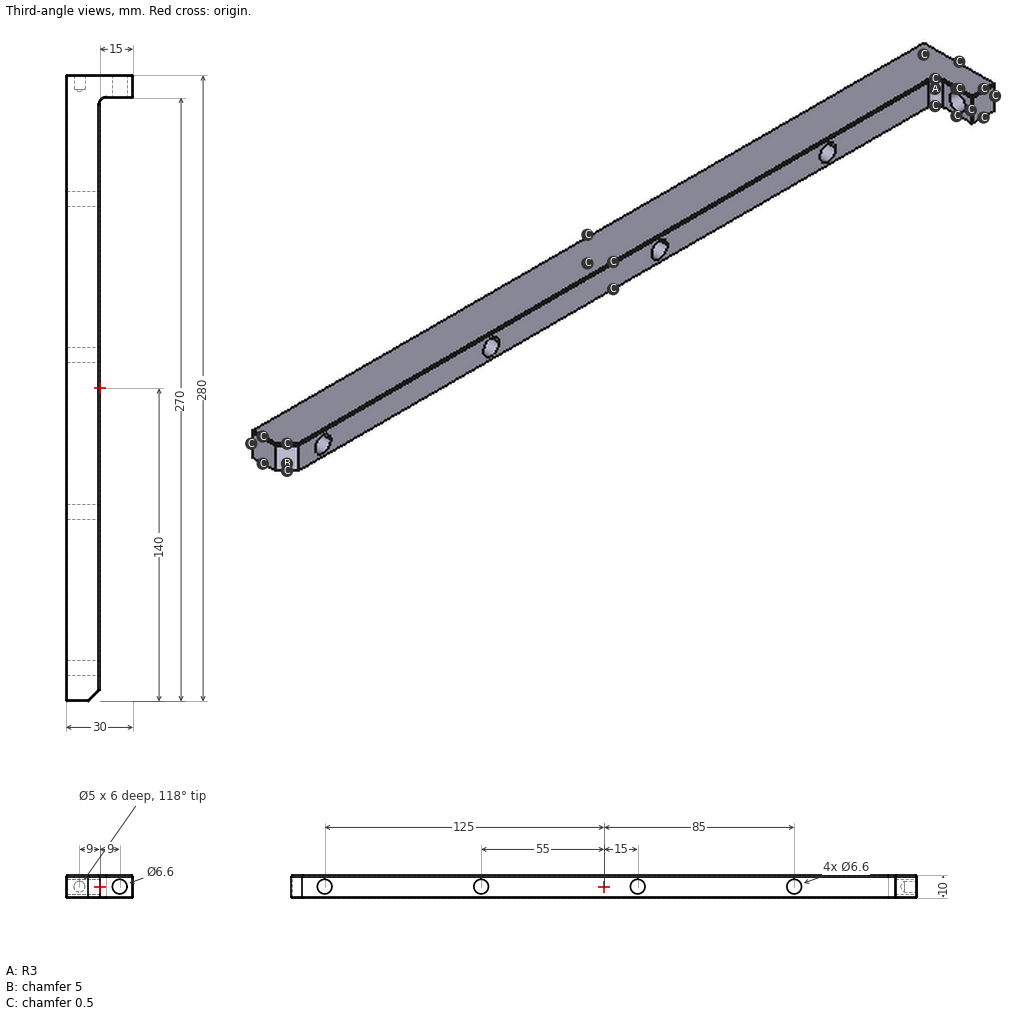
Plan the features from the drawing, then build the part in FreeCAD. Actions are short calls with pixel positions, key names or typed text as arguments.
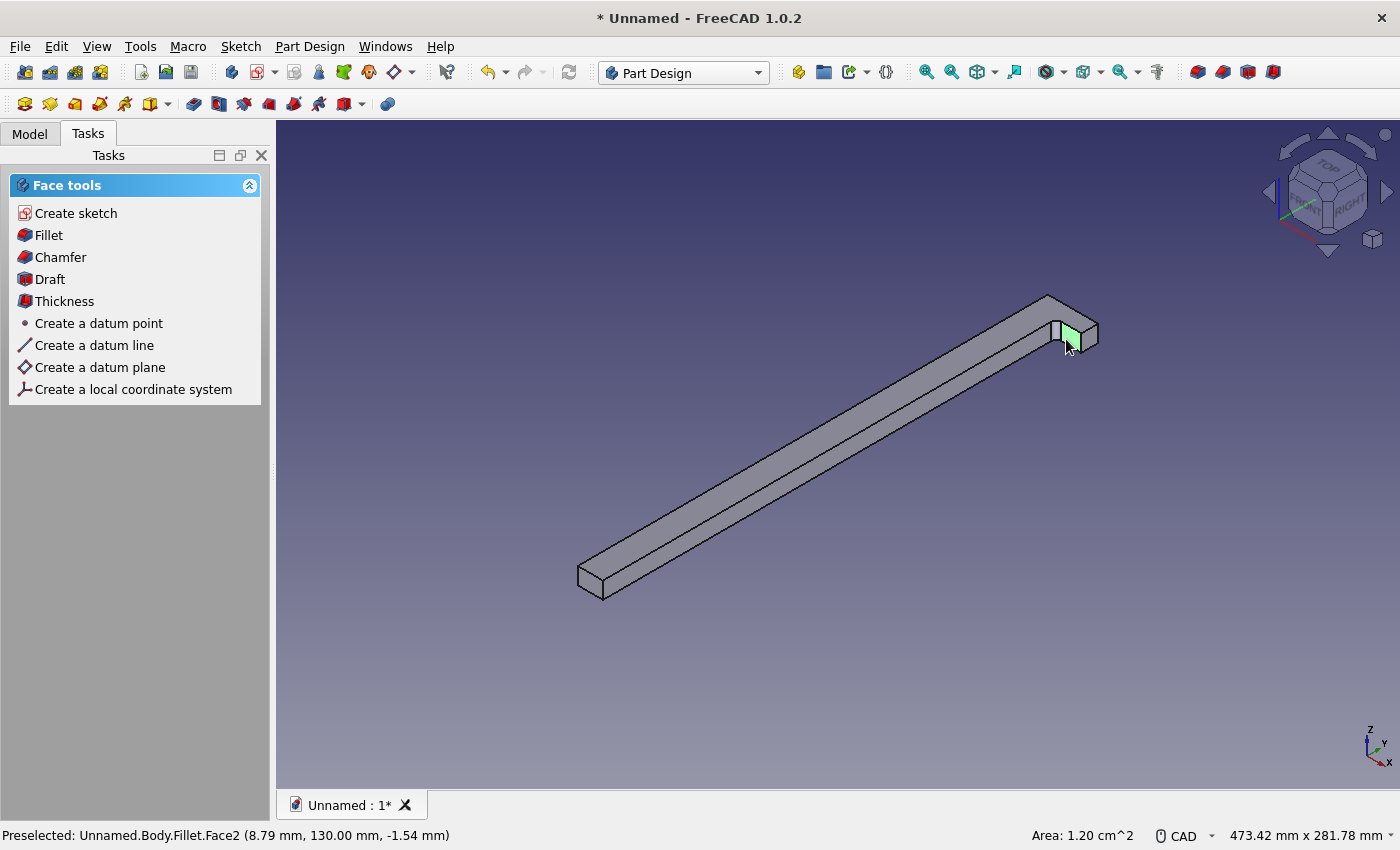
click(256, 72)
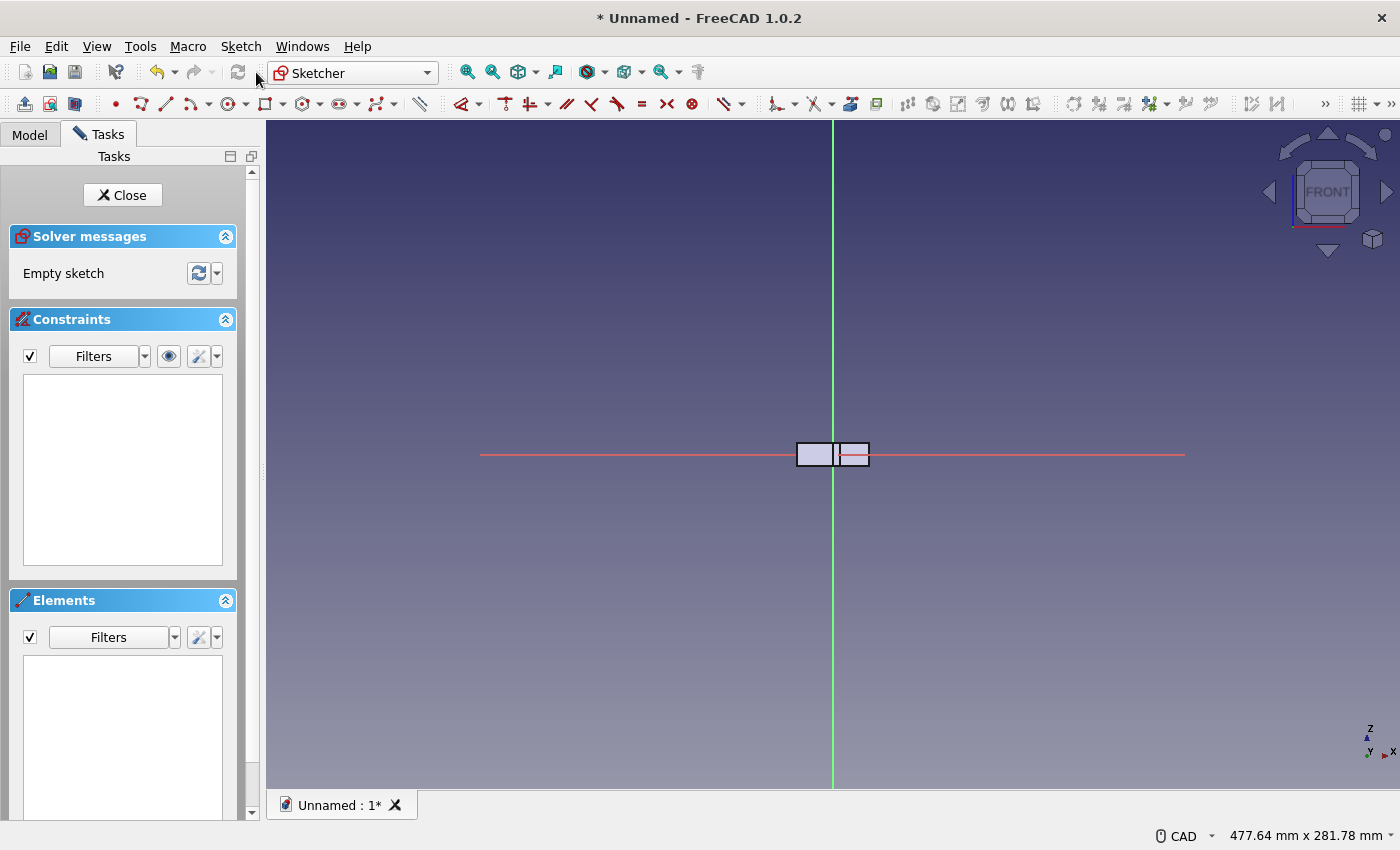
click(75, 104)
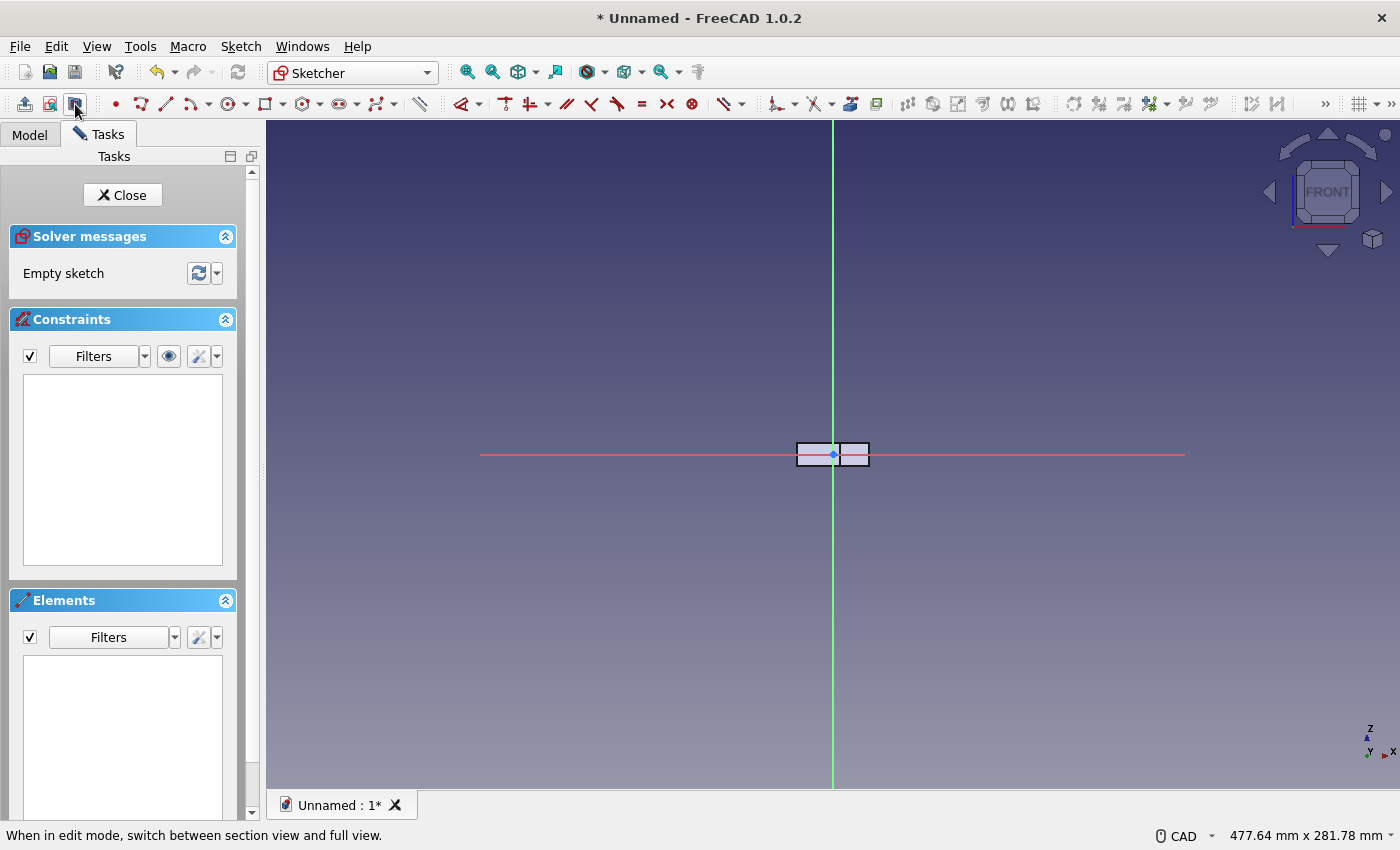
scroll(852, 455, up, 15)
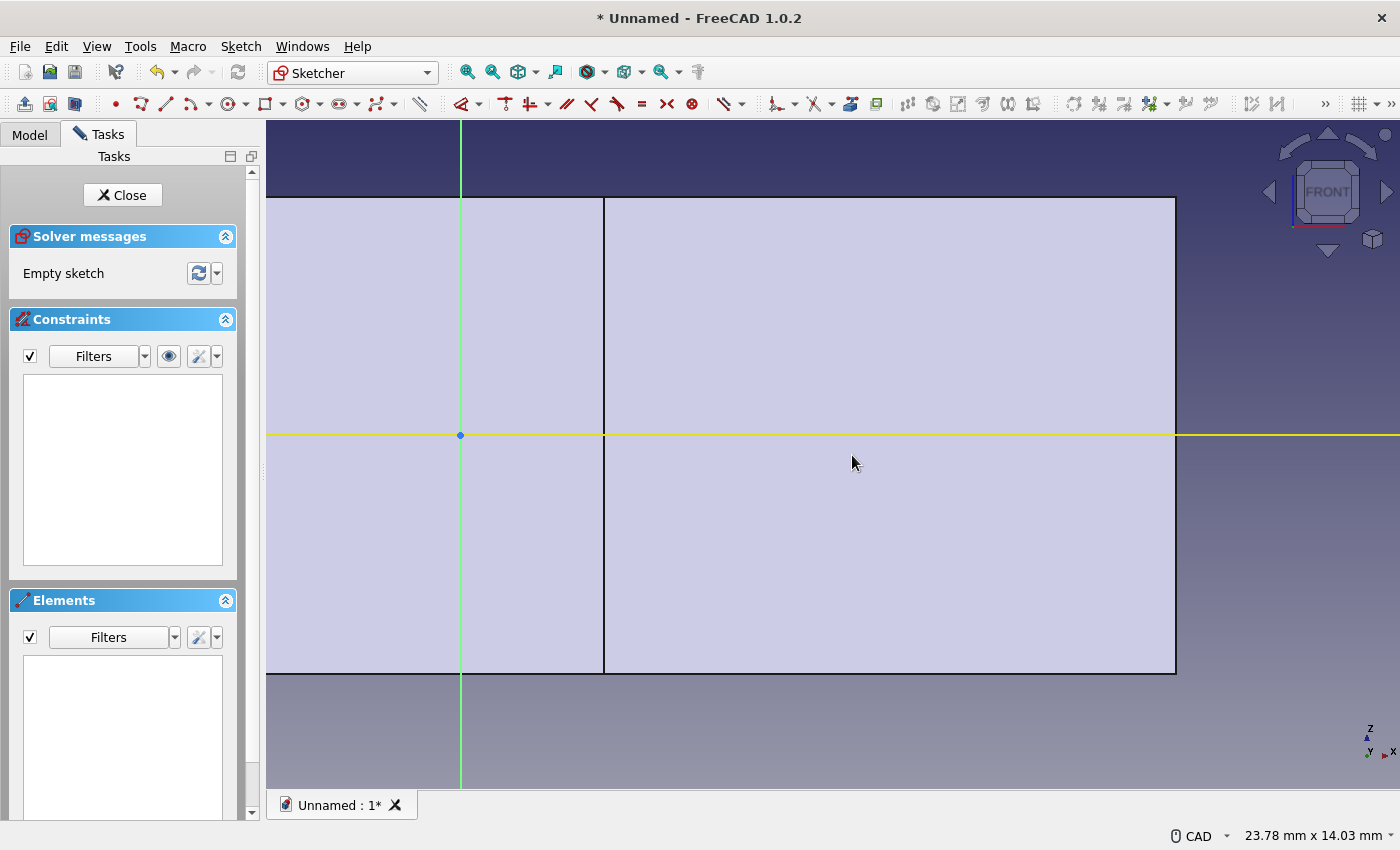
click(228, 104)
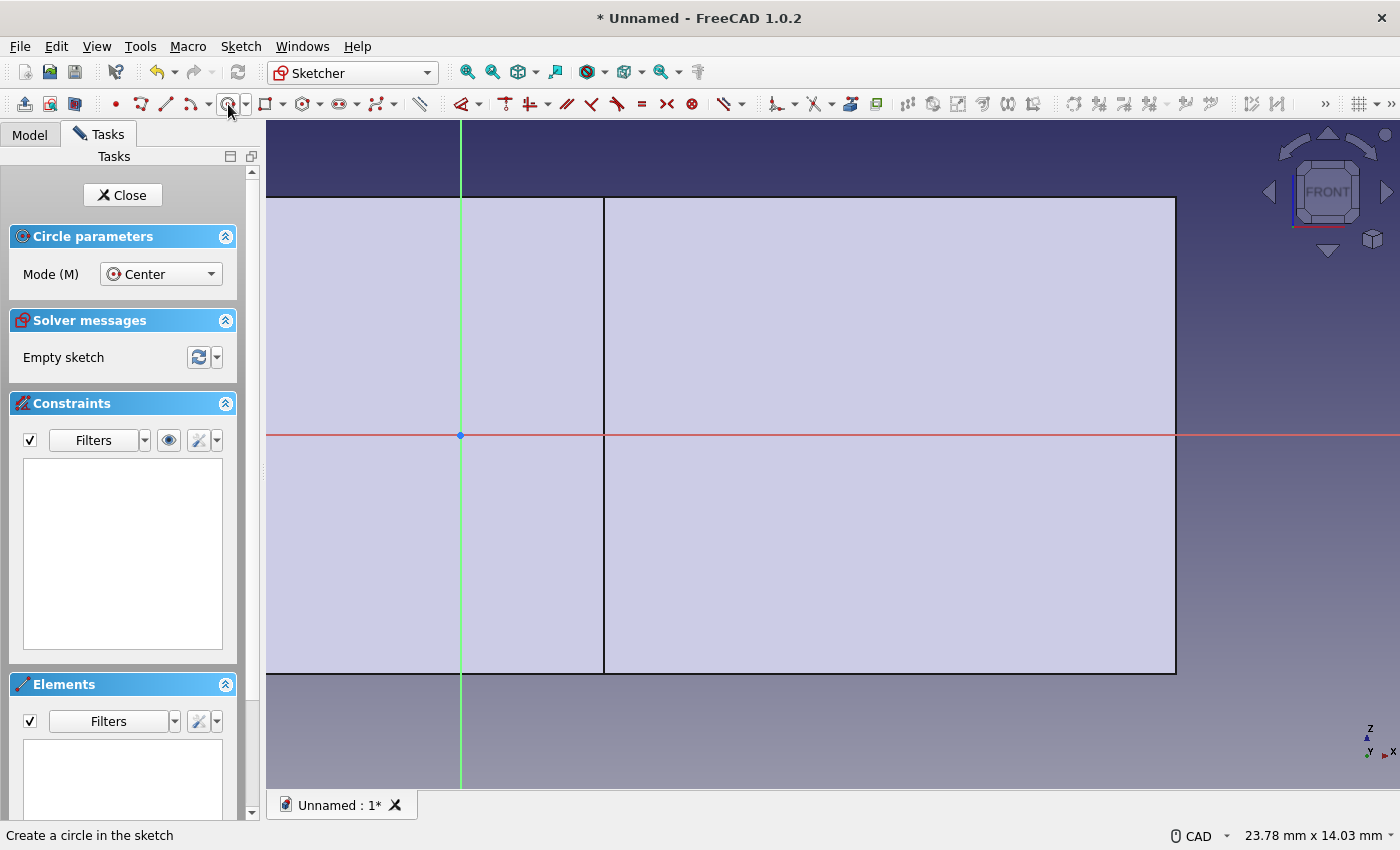
click(890, 435)
click(1001, 324)
key(Escape)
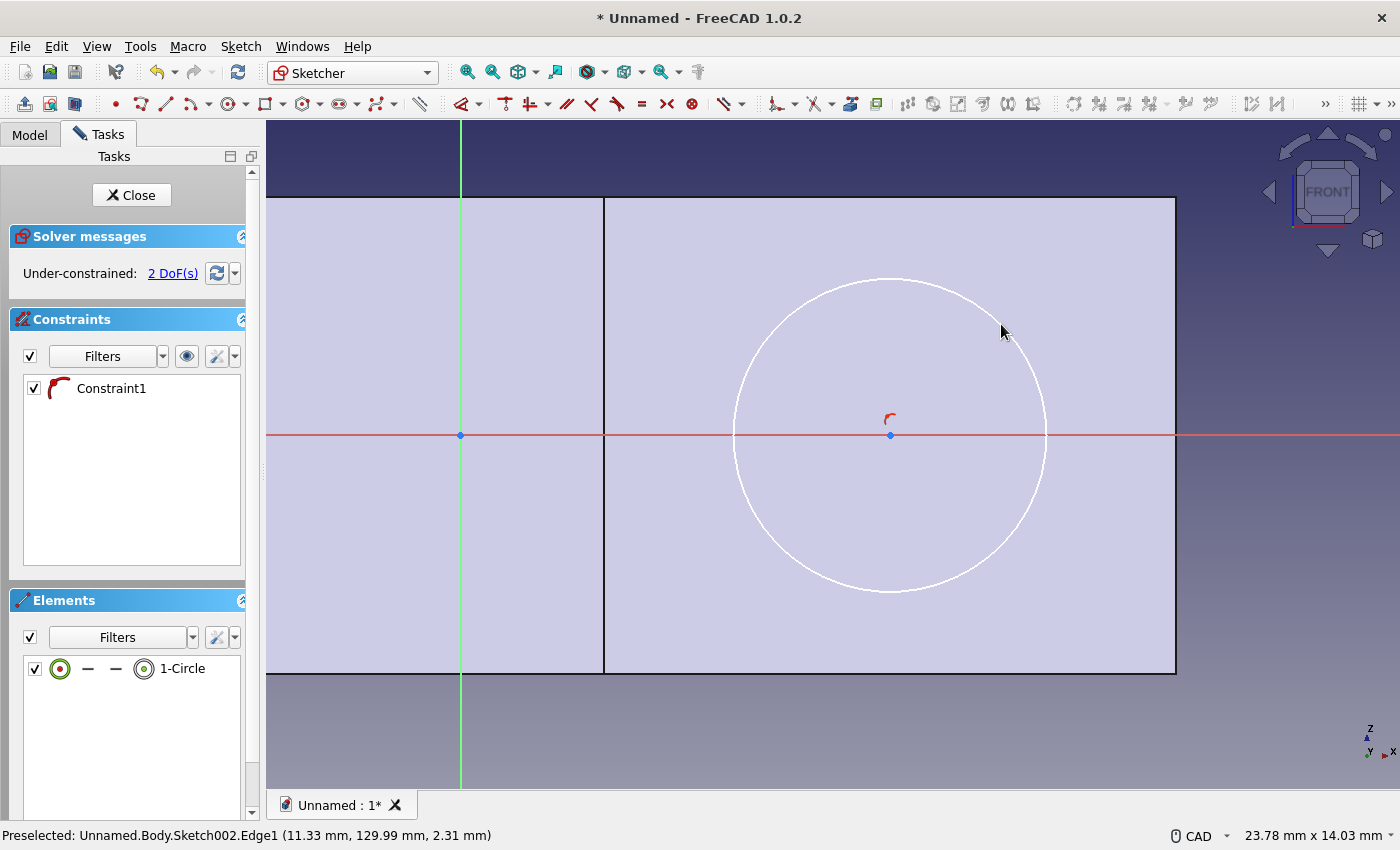
click(460, 104)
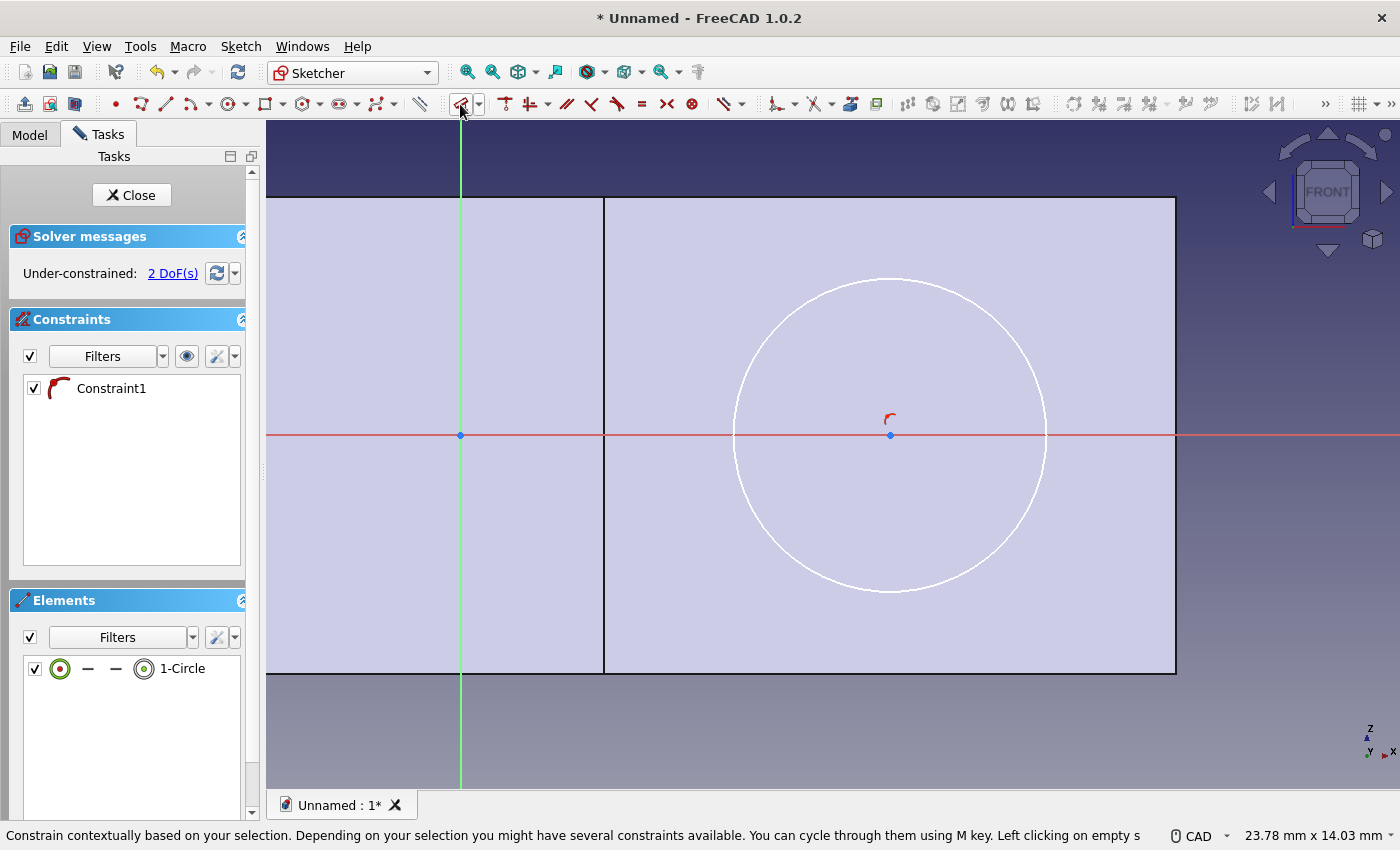
click(1000, 324)
click(1022, 301)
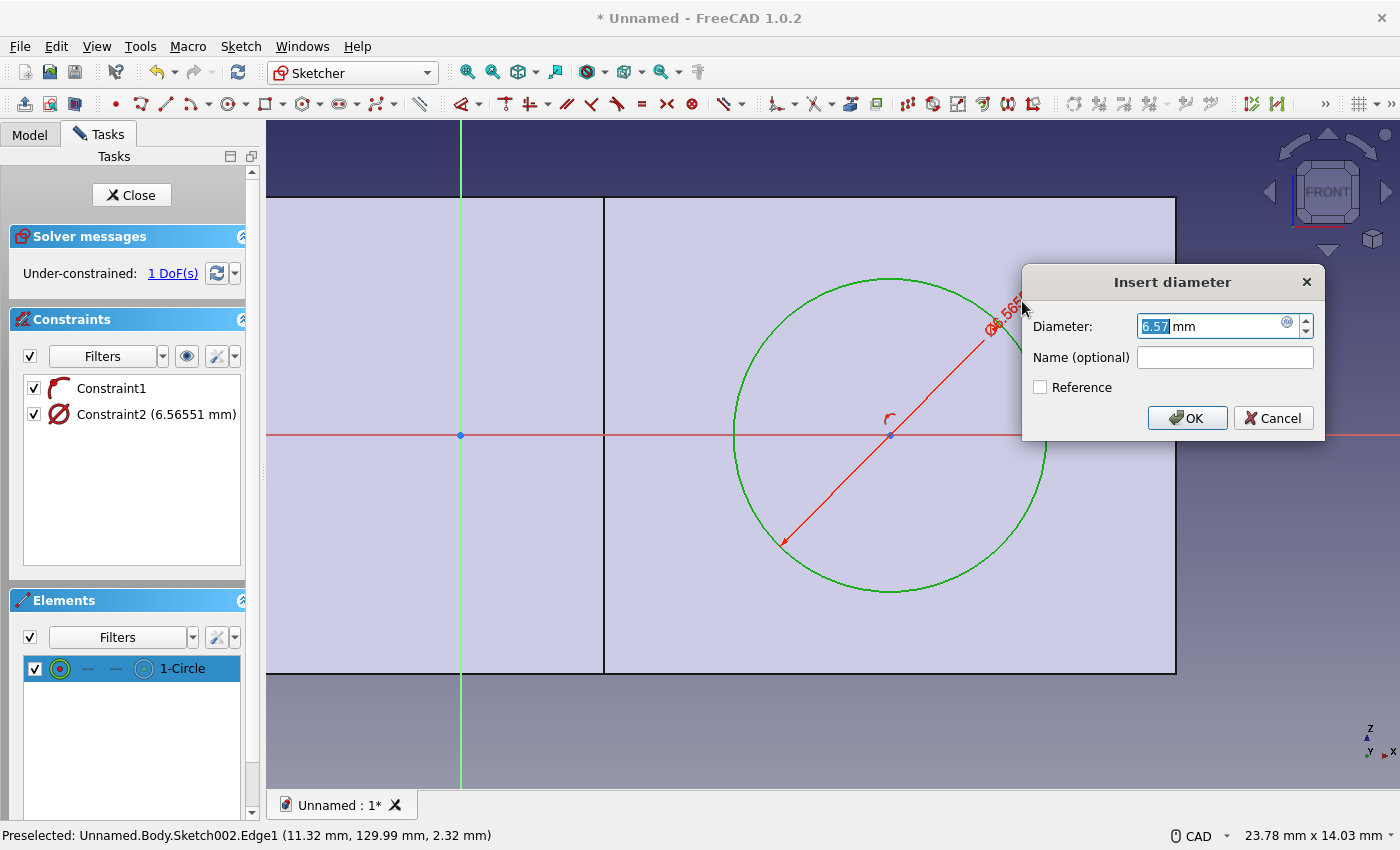
text(6.6)
key(Return)